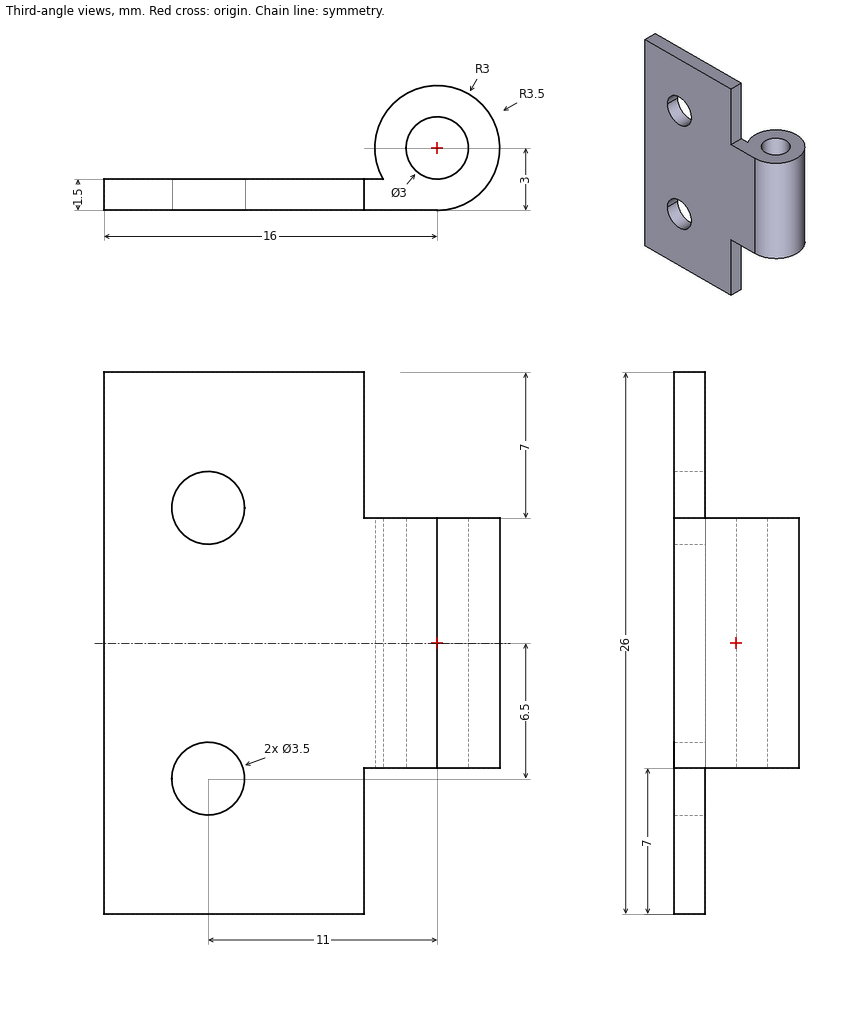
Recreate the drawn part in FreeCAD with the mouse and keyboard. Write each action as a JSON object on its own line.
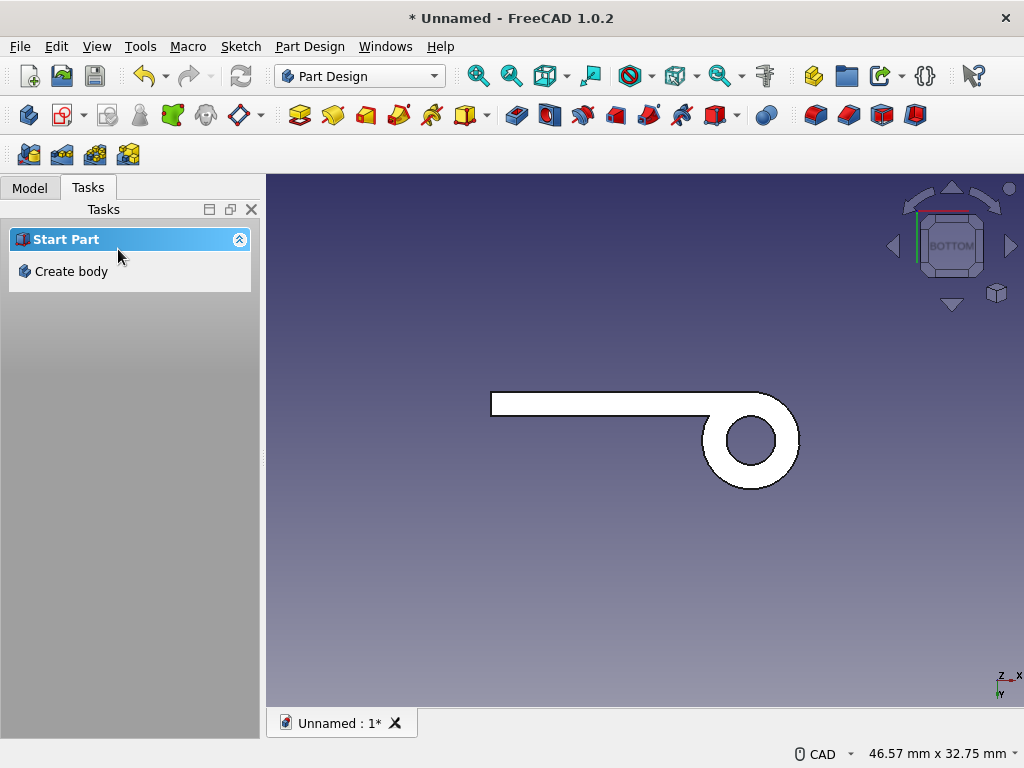
{"action": "left_click", "coordinate": [479, 76]}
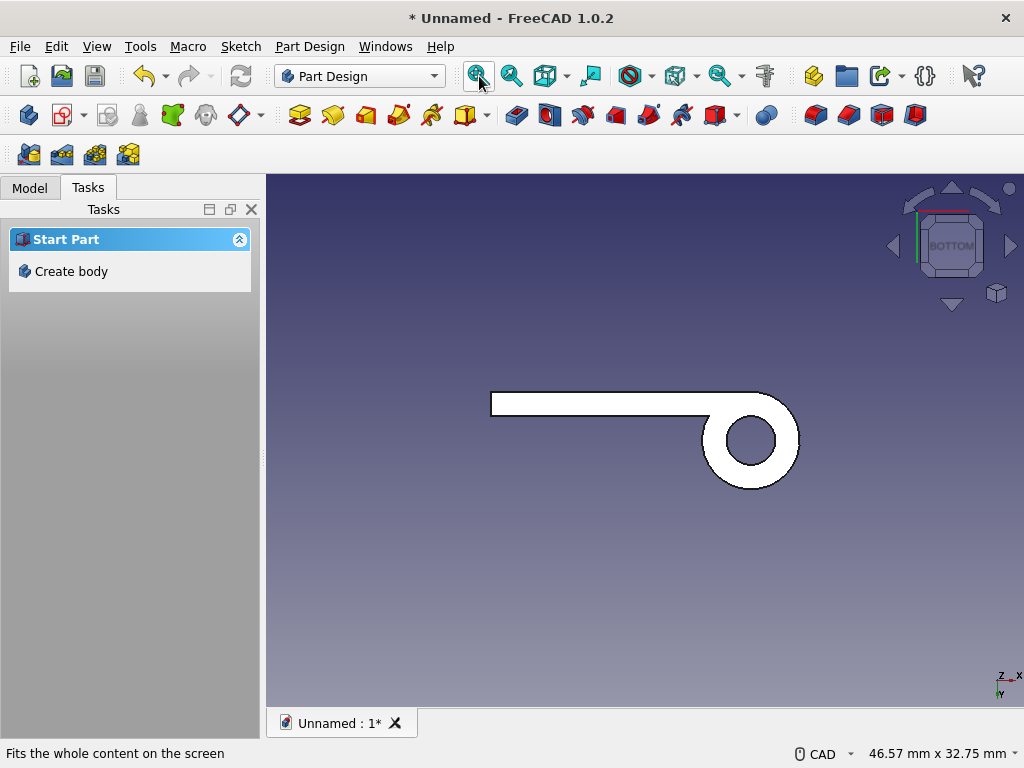
{"action": "left_click", "coordinate": [778, 412]}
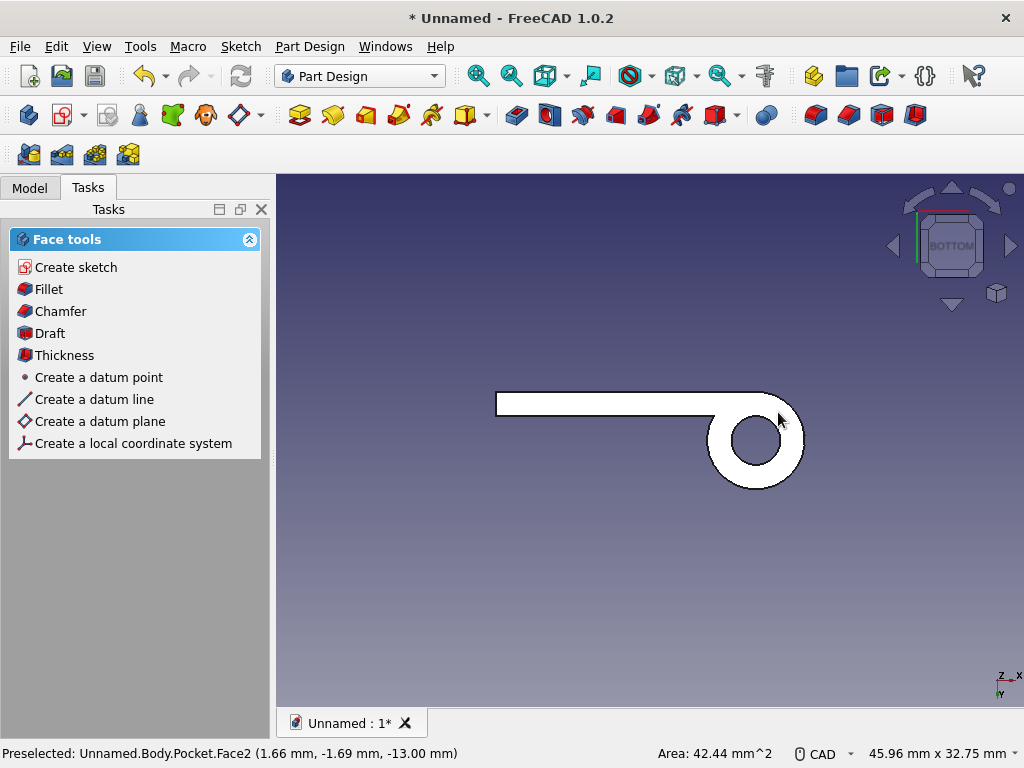
{"action": "left_click", "coordinate": [62, 116]}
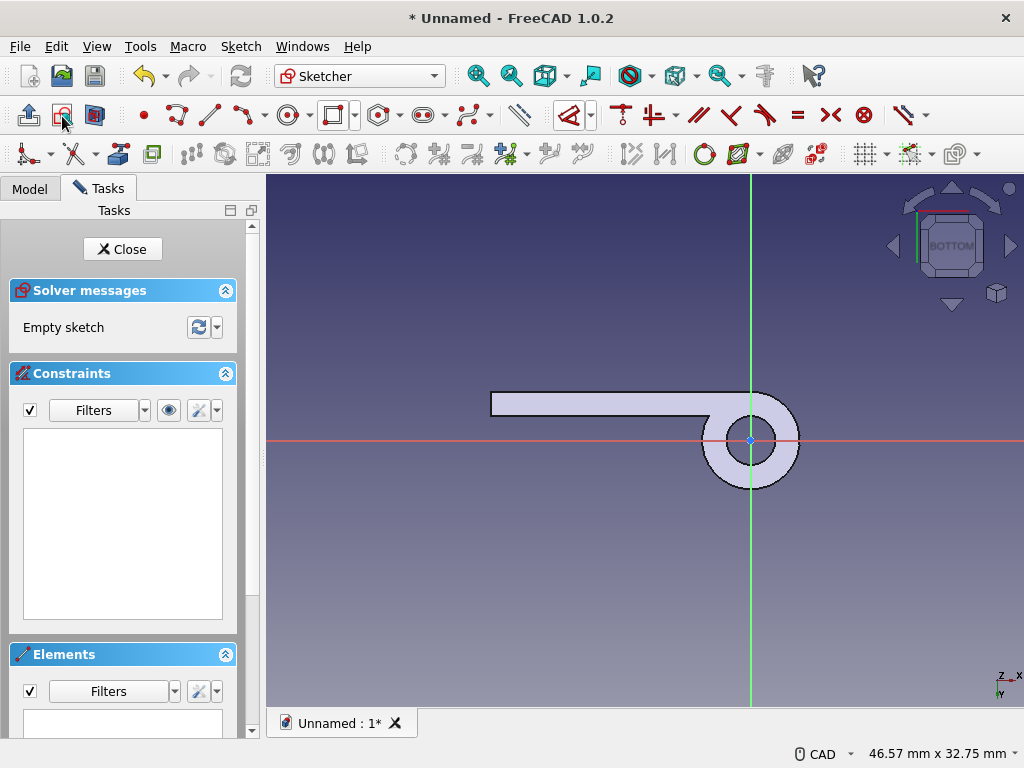
{"action": "scroll", "coordinate": [803, 427], "scroll_direction": "up", "scroll_amount": 7}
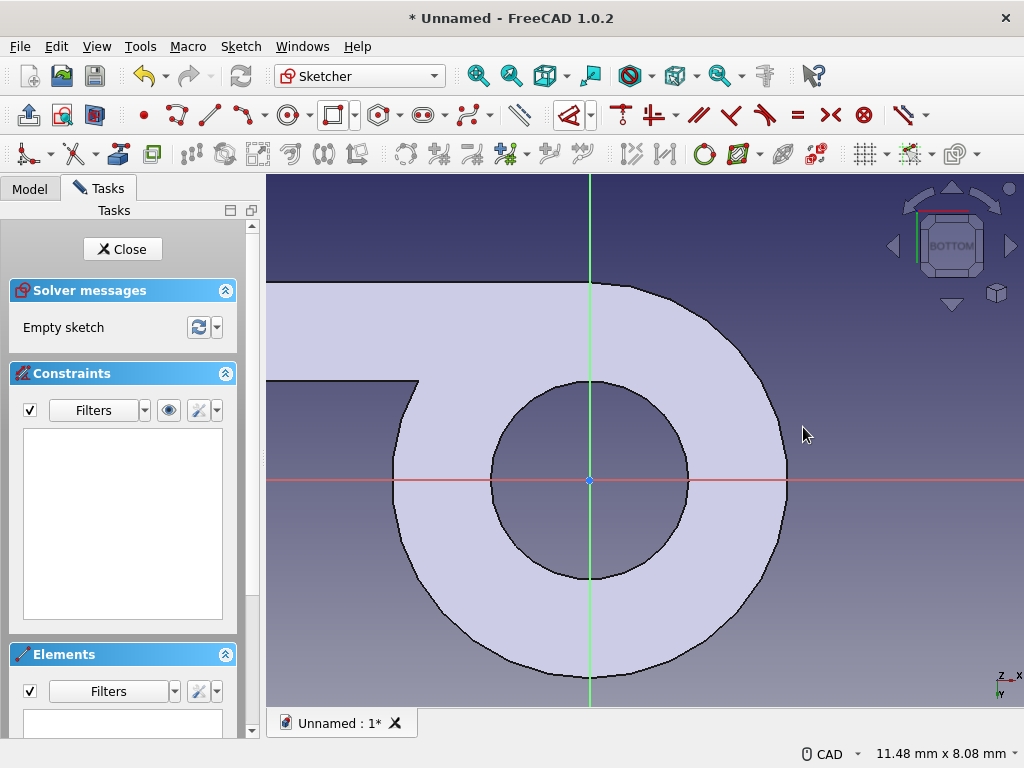
{"action": "left_click", "coordinate": [177, 116]}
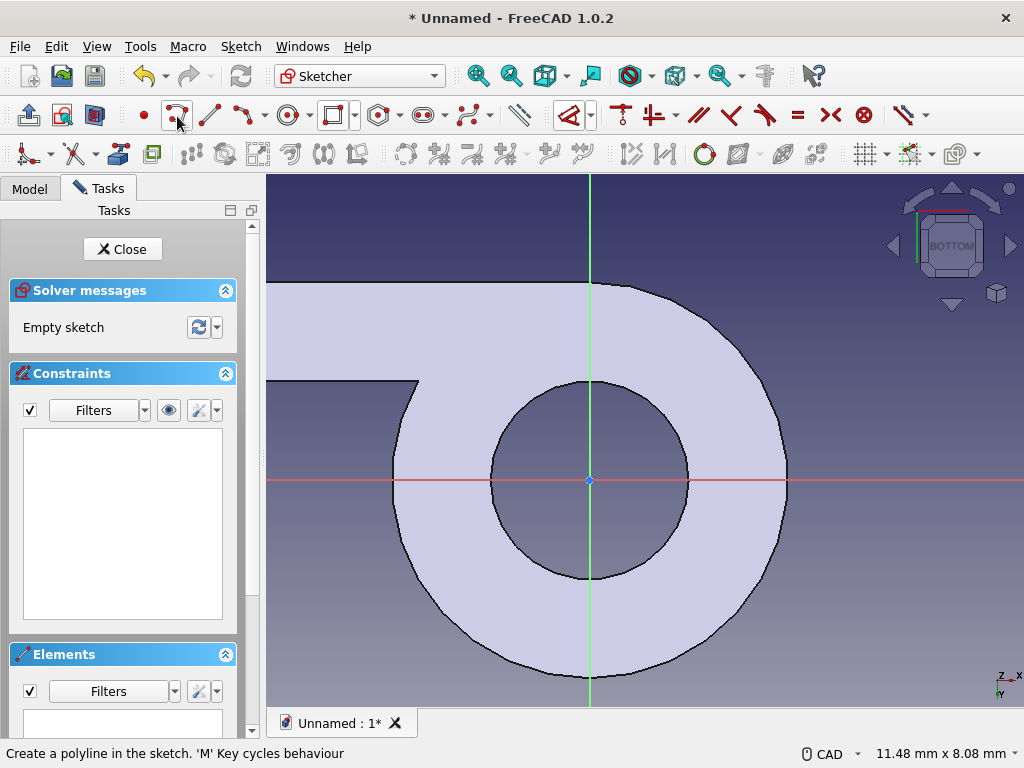
{"action": "left_click", "coordinate": [471, 282]}
{"action": "left_click", "coordinate": [359, 282]}
{"action": "left_click", "coordinate": [359, 480]}
{"action": "right_click", "coordinate": [359, 480]}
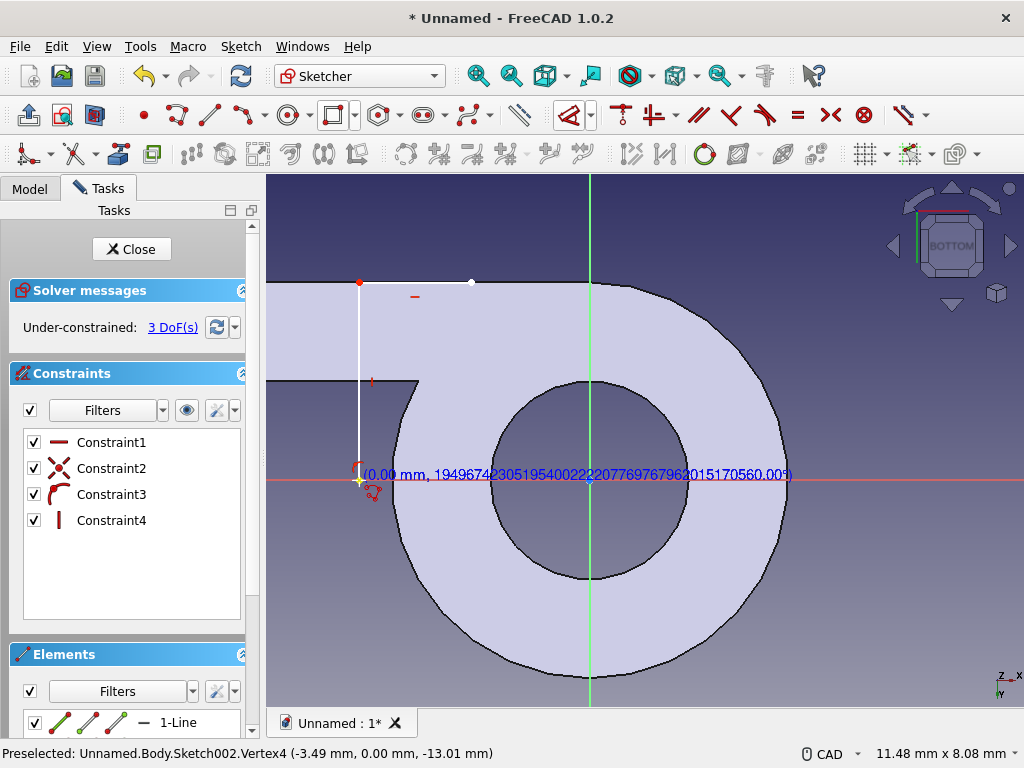
{"action": "left_click", "coordinate": [242, 116]}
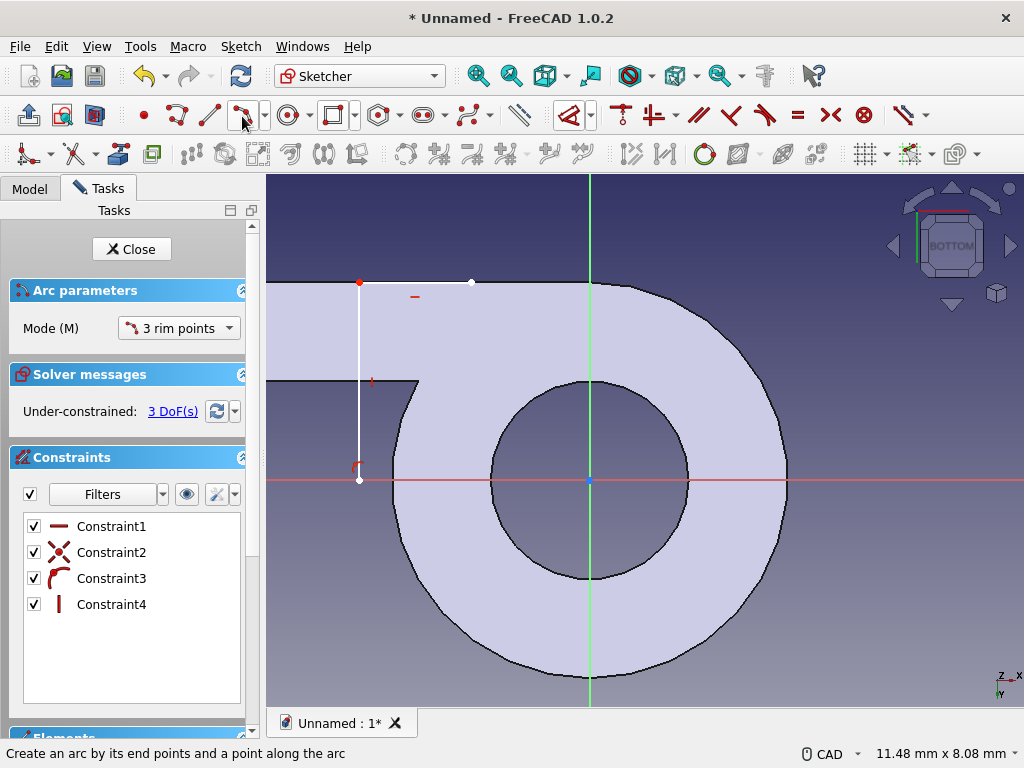
{"action": "left_click", "coordinate": [359, 480]}
{"action": "left_click", "coordinate": [471, 283]}
{"action": "left_click", "coordinate": [791, 594]}
{"action": "key", "text": "Escape"}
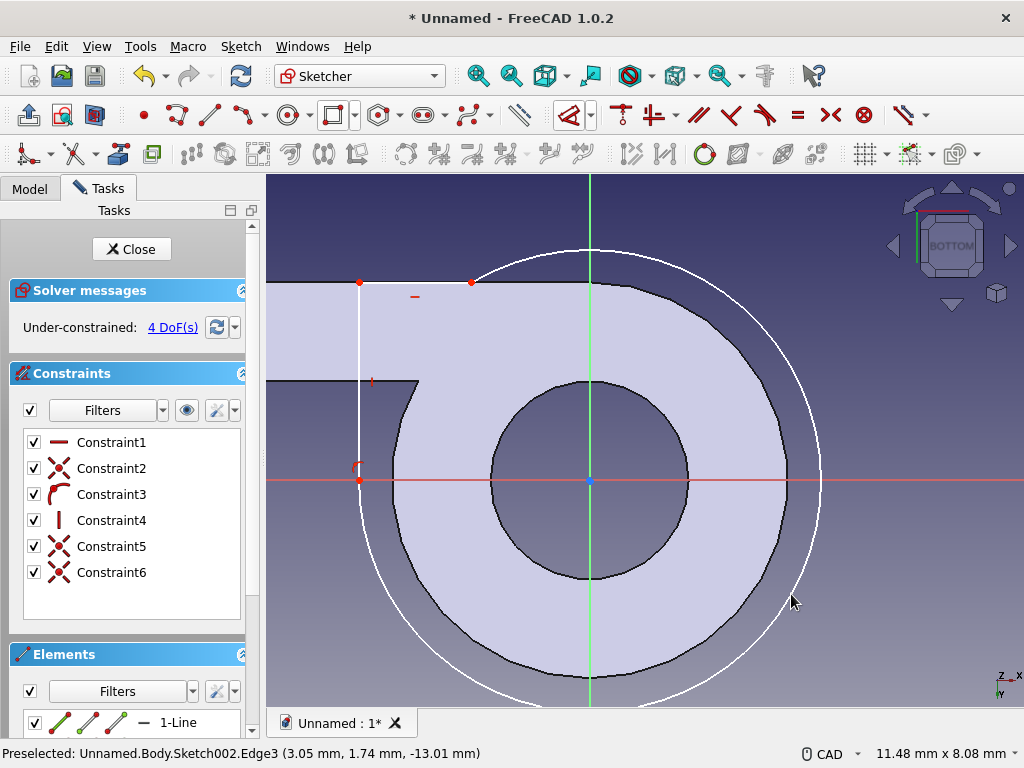
{"action": "left_click", "coordinate": [359, 342]}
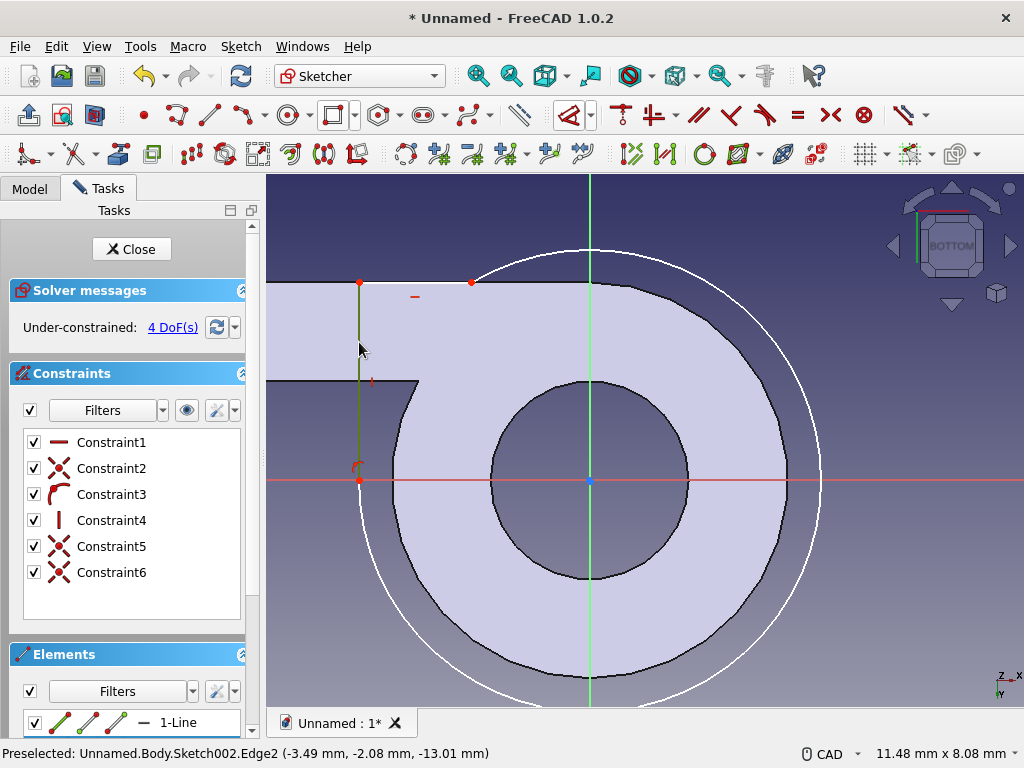
{"action": "left_click", "coordinate": [789, 363]}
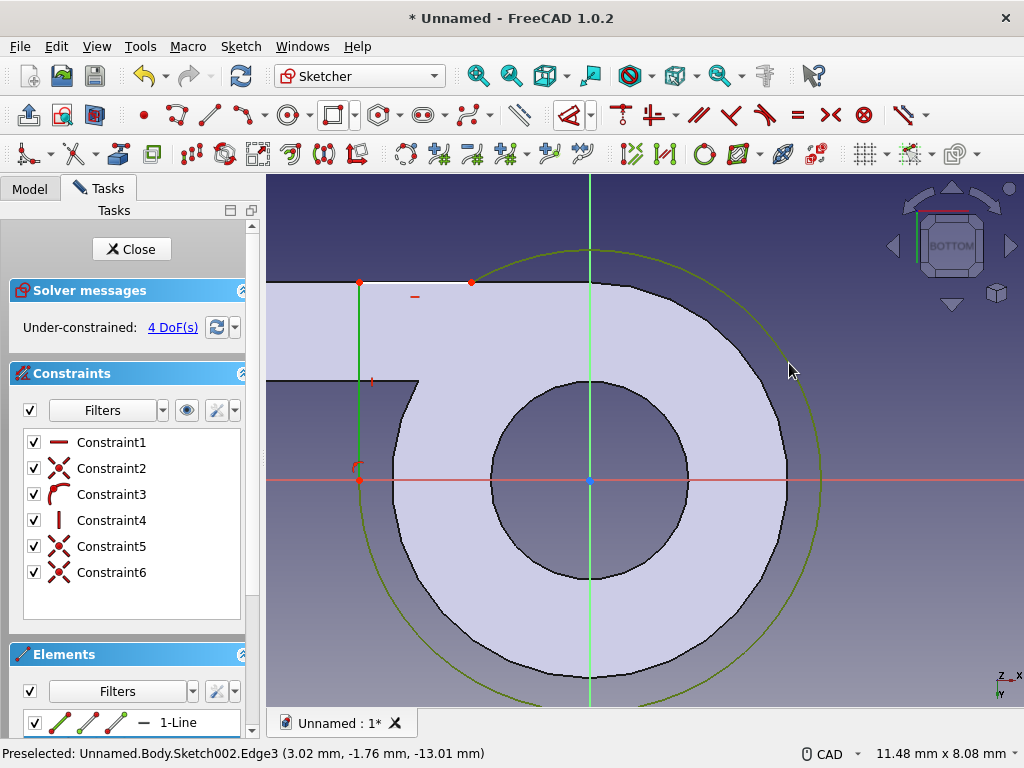
{"action": "left_click", "coordinate": [765, 116]}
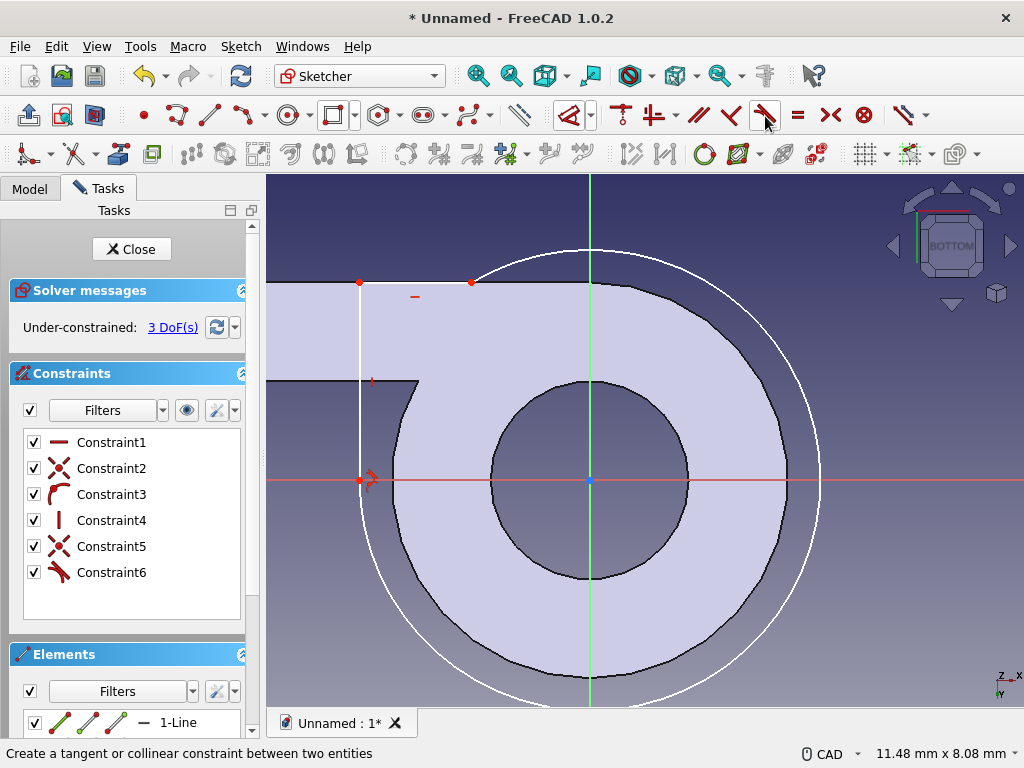
{"action": "left_click", "coordinate": [590, 480]}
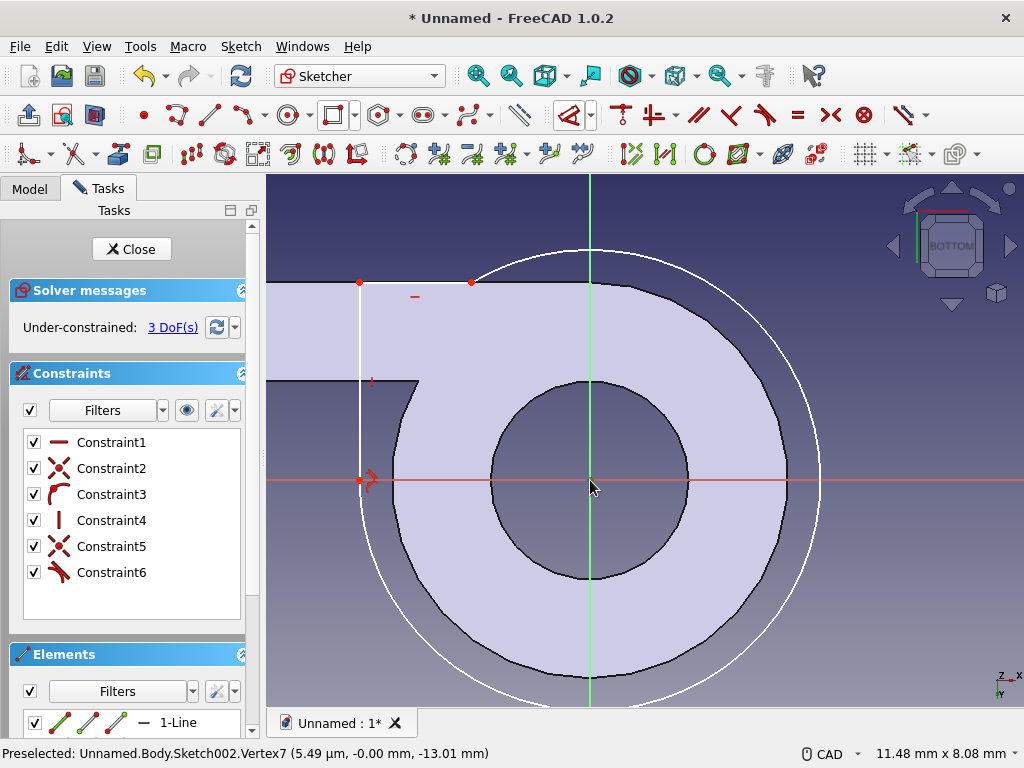
{"action": "left_click", "coordinate": [590, 645]}